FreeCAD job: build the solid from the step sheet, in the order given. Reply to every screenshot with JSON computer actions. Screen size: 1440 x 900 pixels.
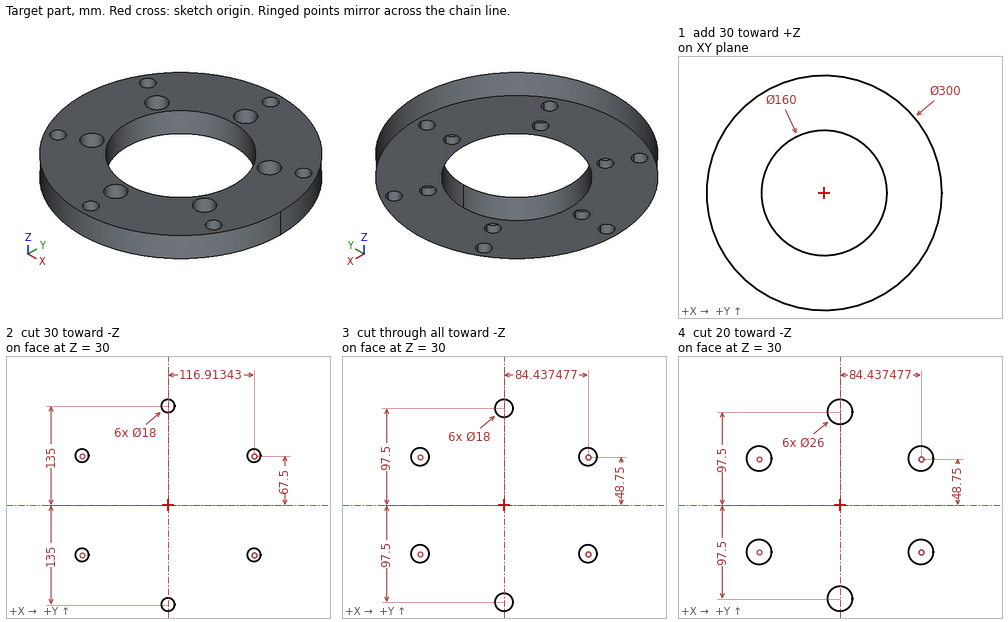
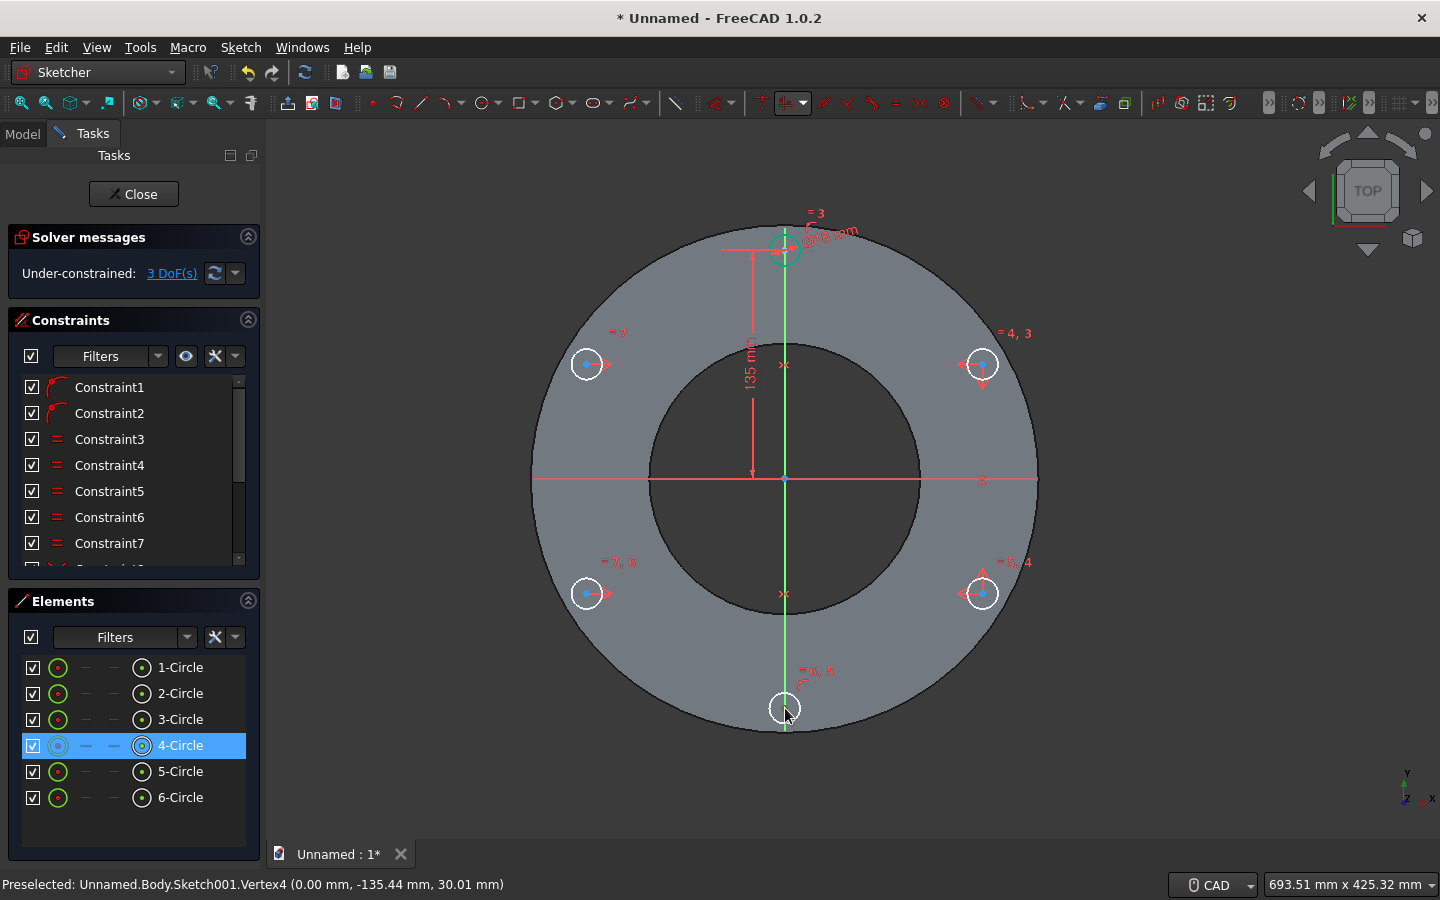
{"action": "key", "text": "i"}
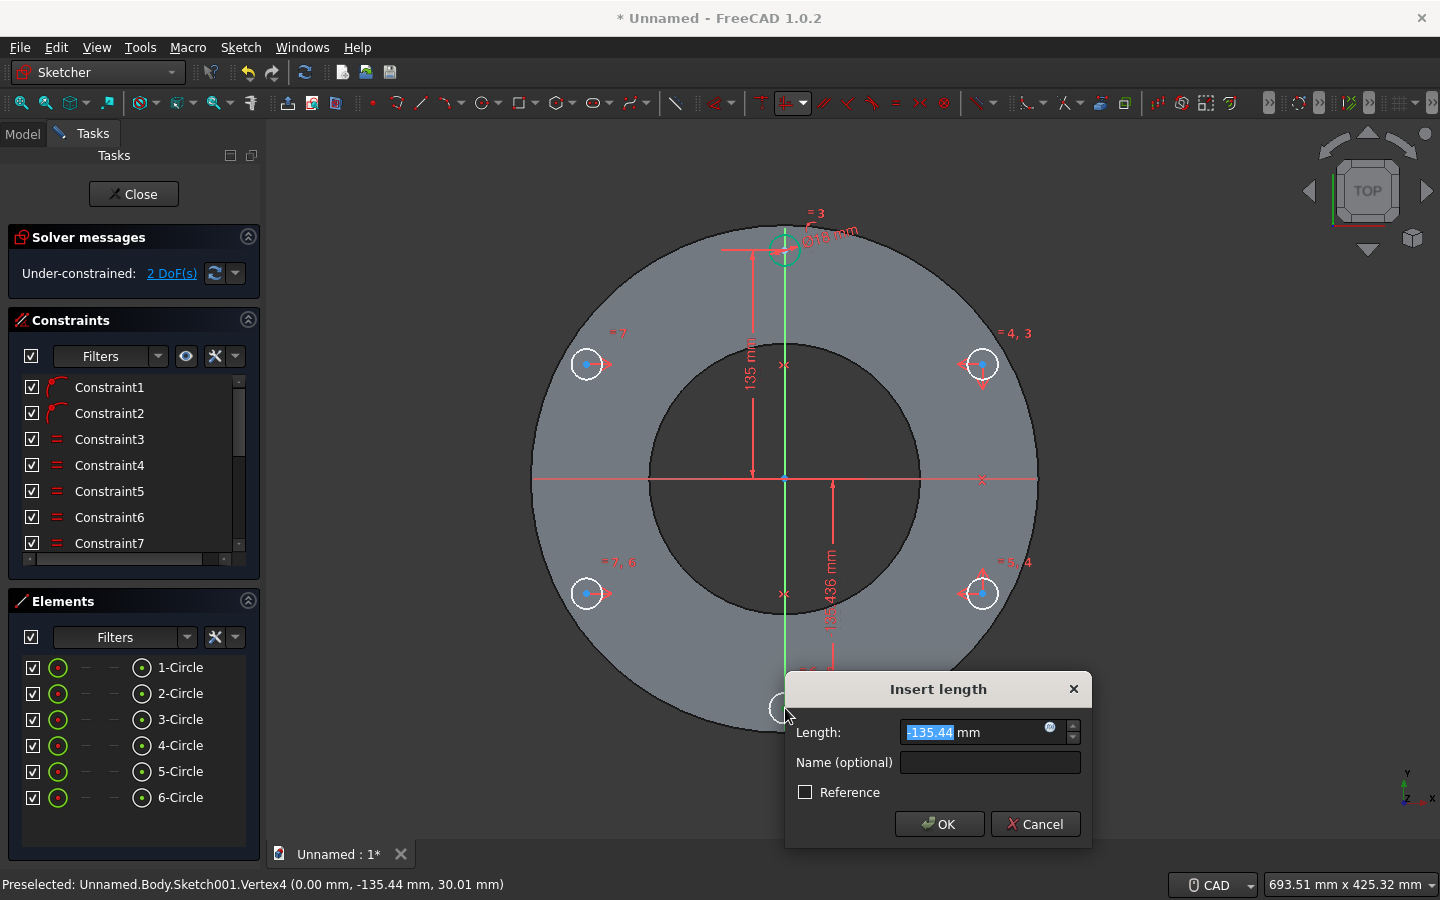
{"action": "type", "text": "-135"}
{"action": "key", "text": "Return"}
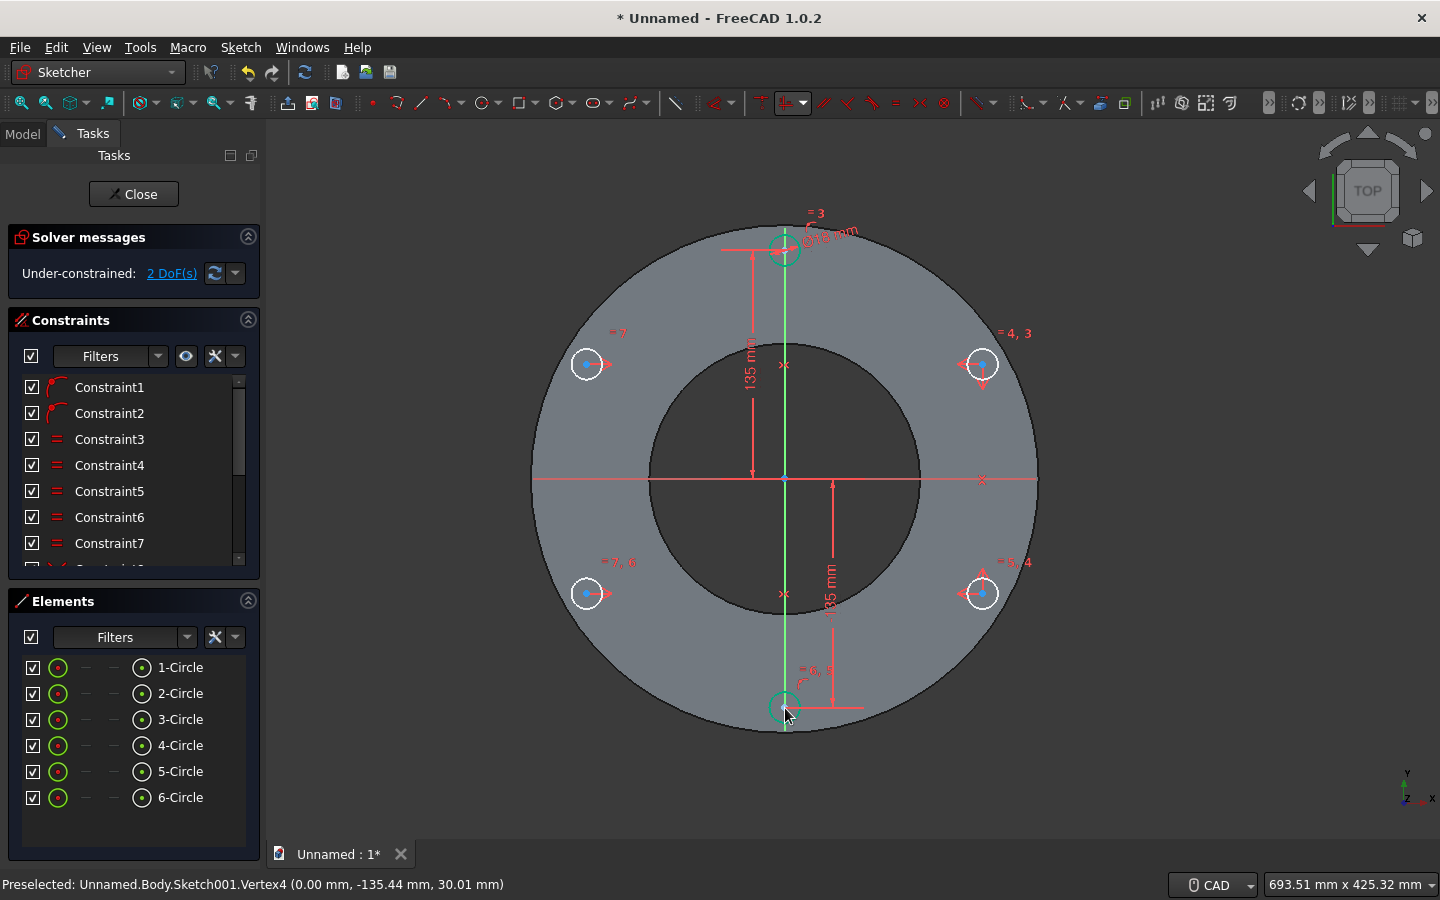
{"action": "left_click", "coordinate": [983, 364]}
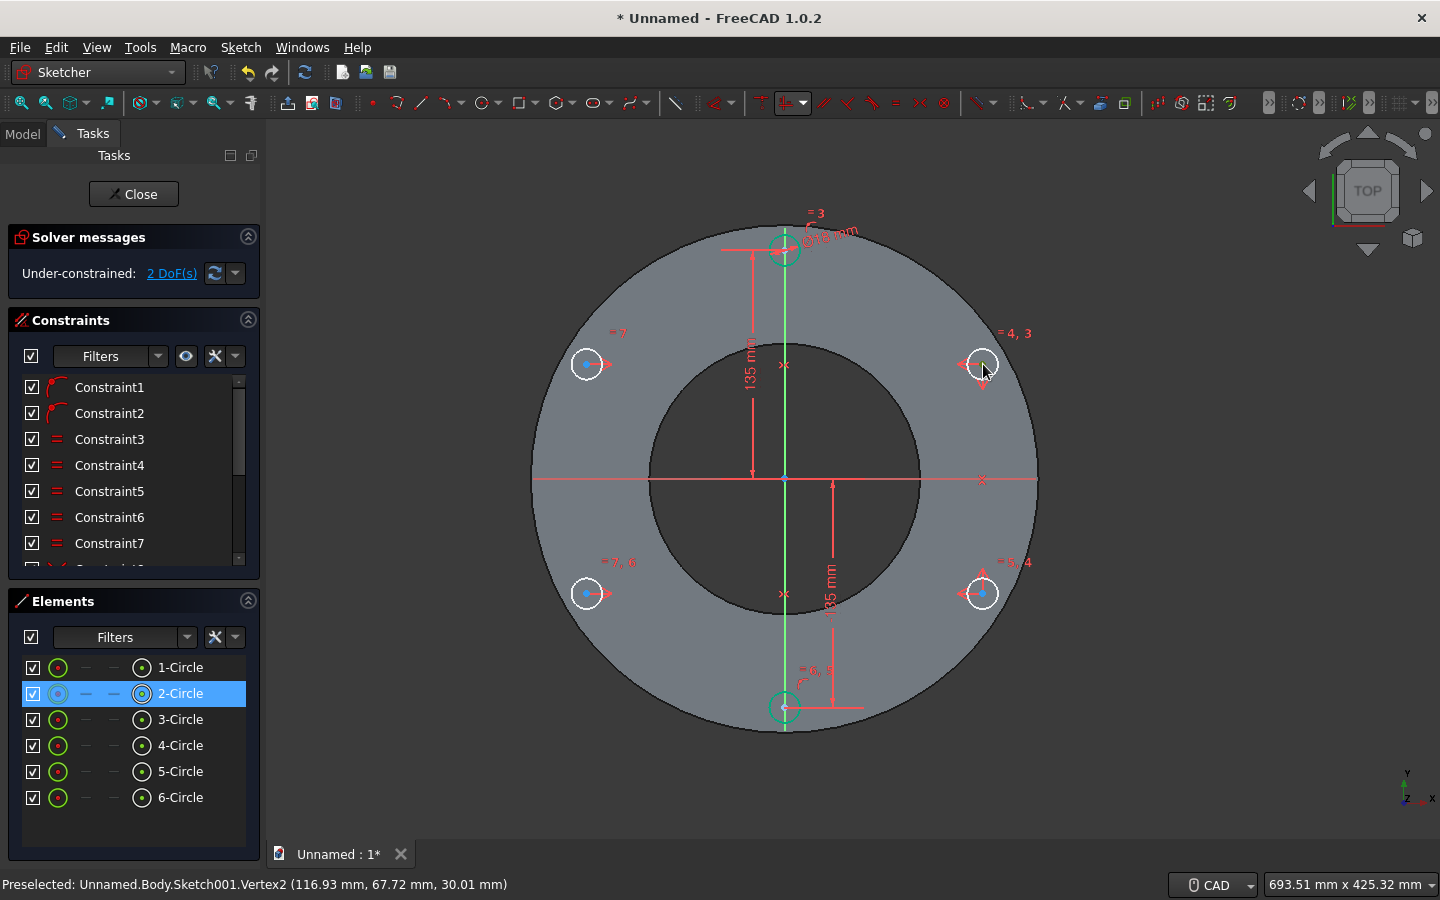
{"action": "key", "text": "i"}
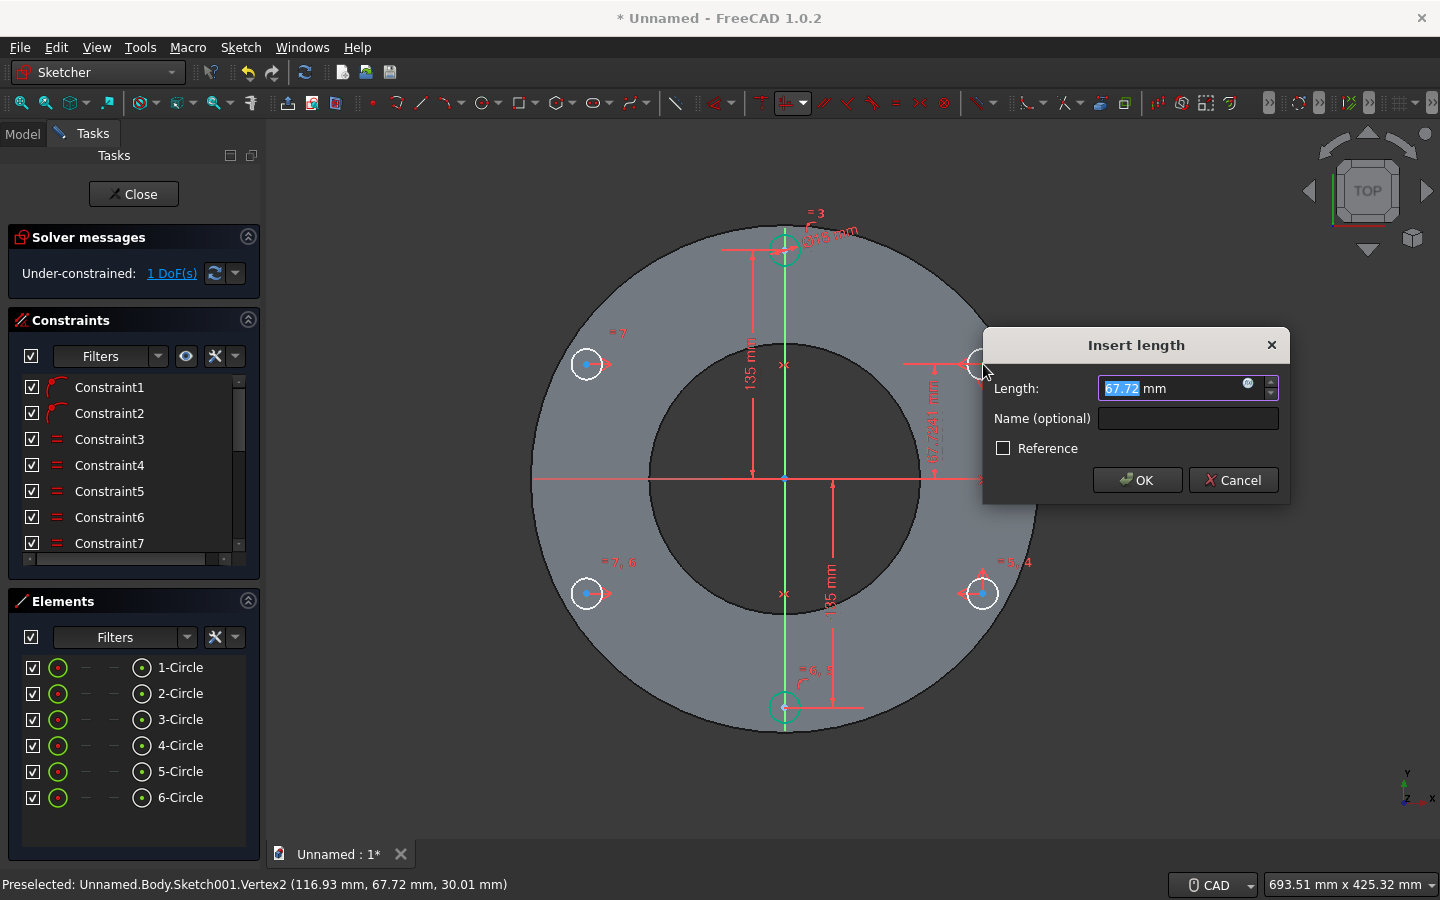
{"action": "type", "text": "67.5"}
{"action": "key", "text": "Return"}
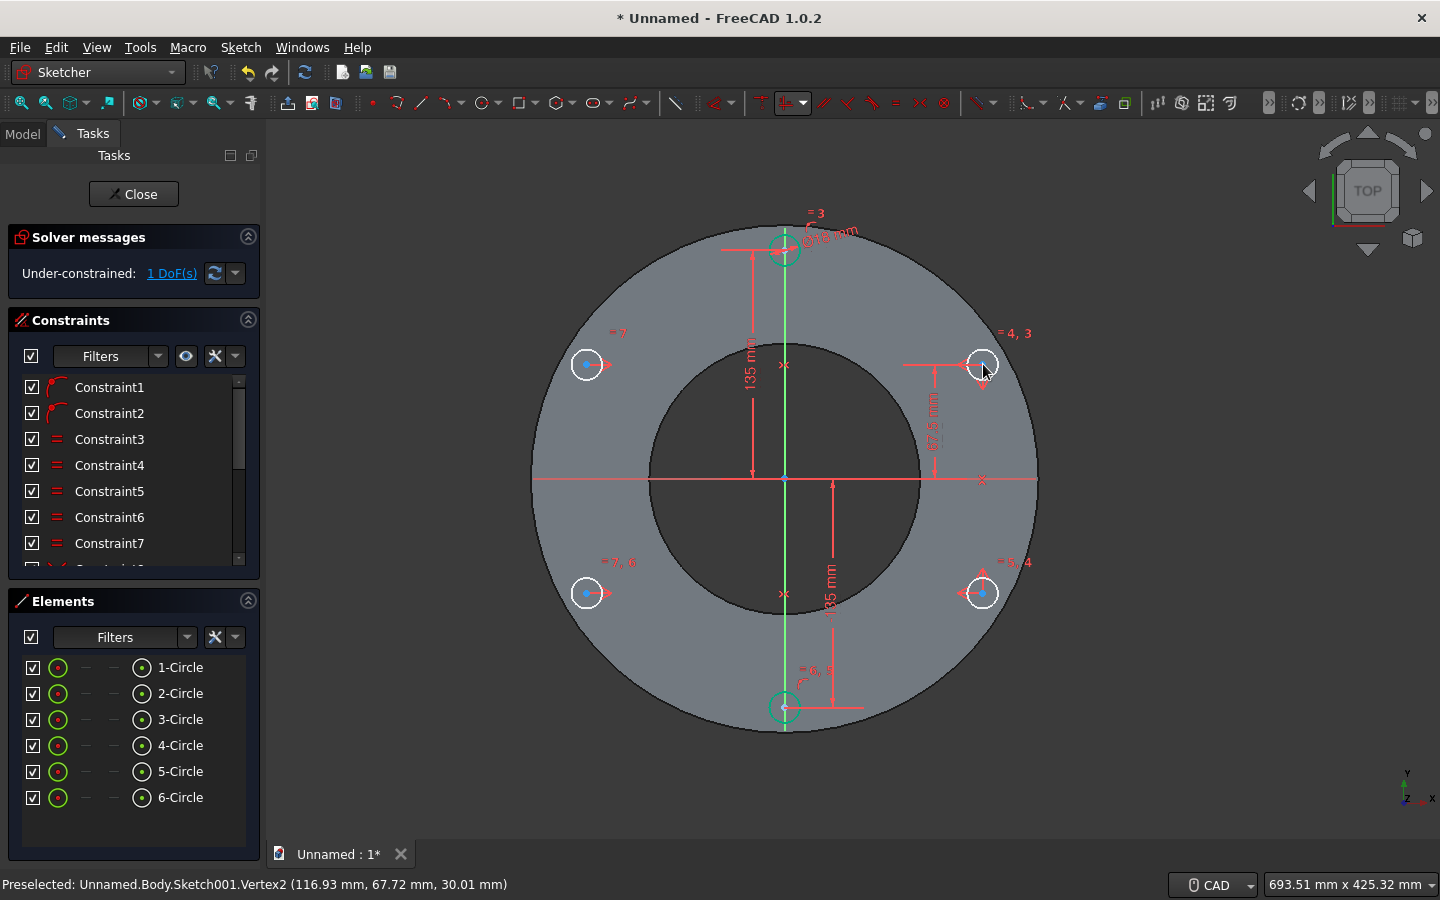
{"action": "left_click", "coordinate": [983, 365]}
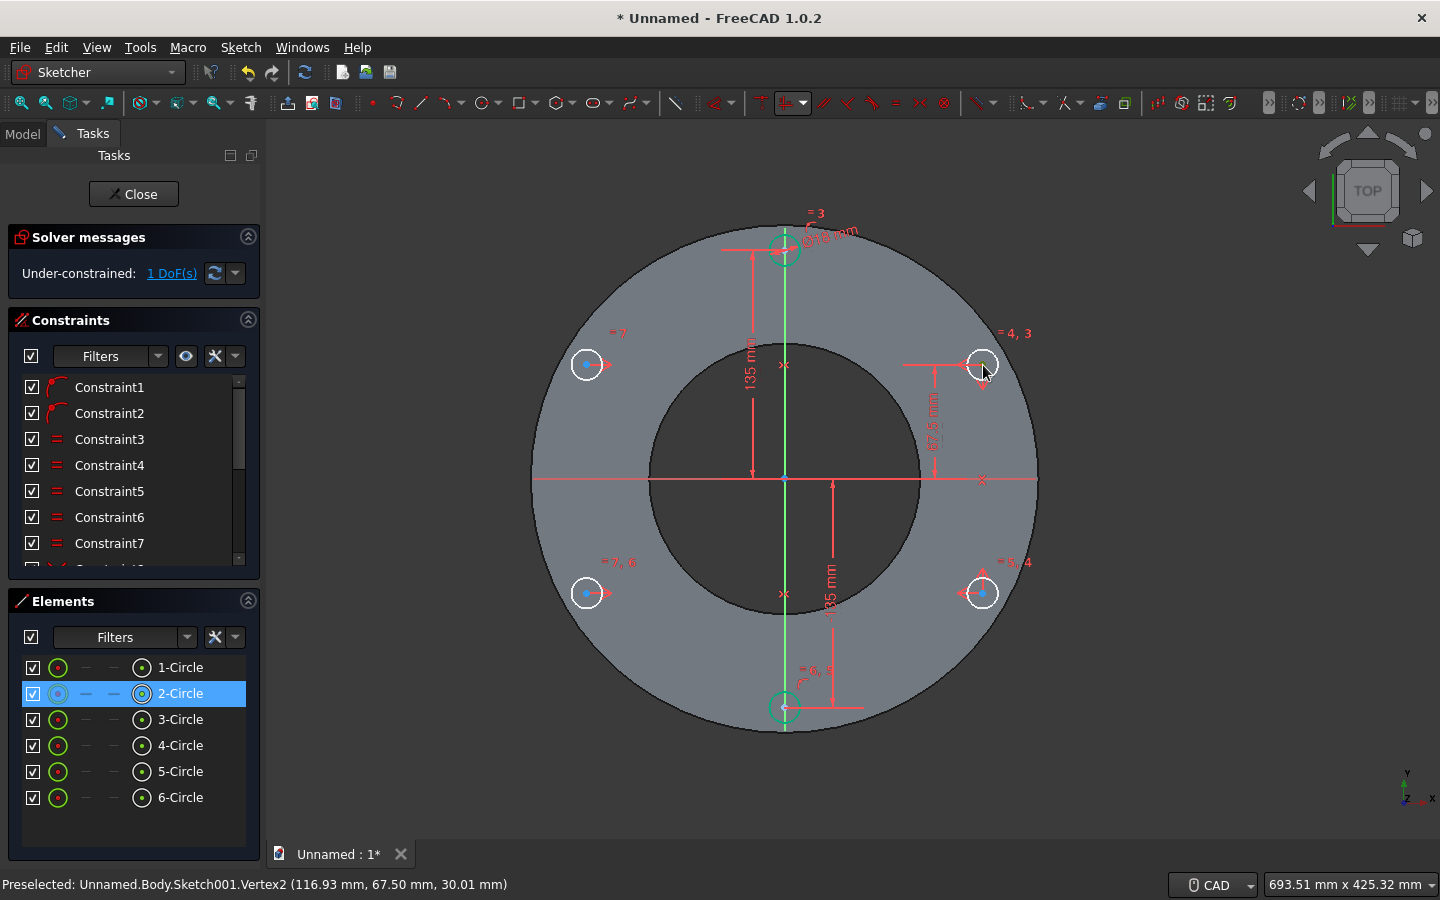
{"action": "key", "text": "l"}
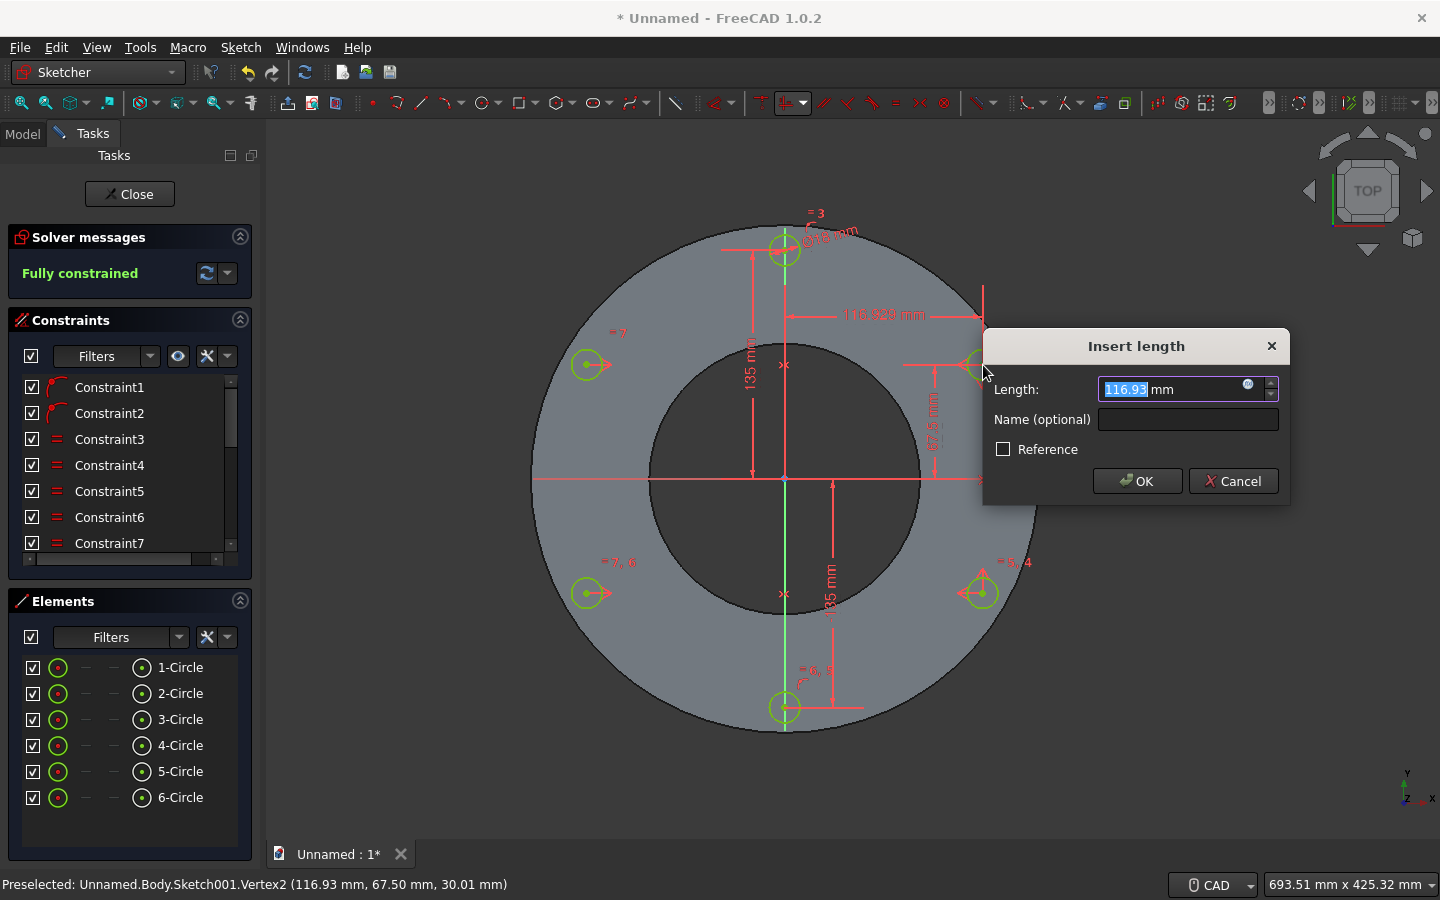
{"action": "type", "text": "116.91343"}
{"action": "key", "text": "Return"}